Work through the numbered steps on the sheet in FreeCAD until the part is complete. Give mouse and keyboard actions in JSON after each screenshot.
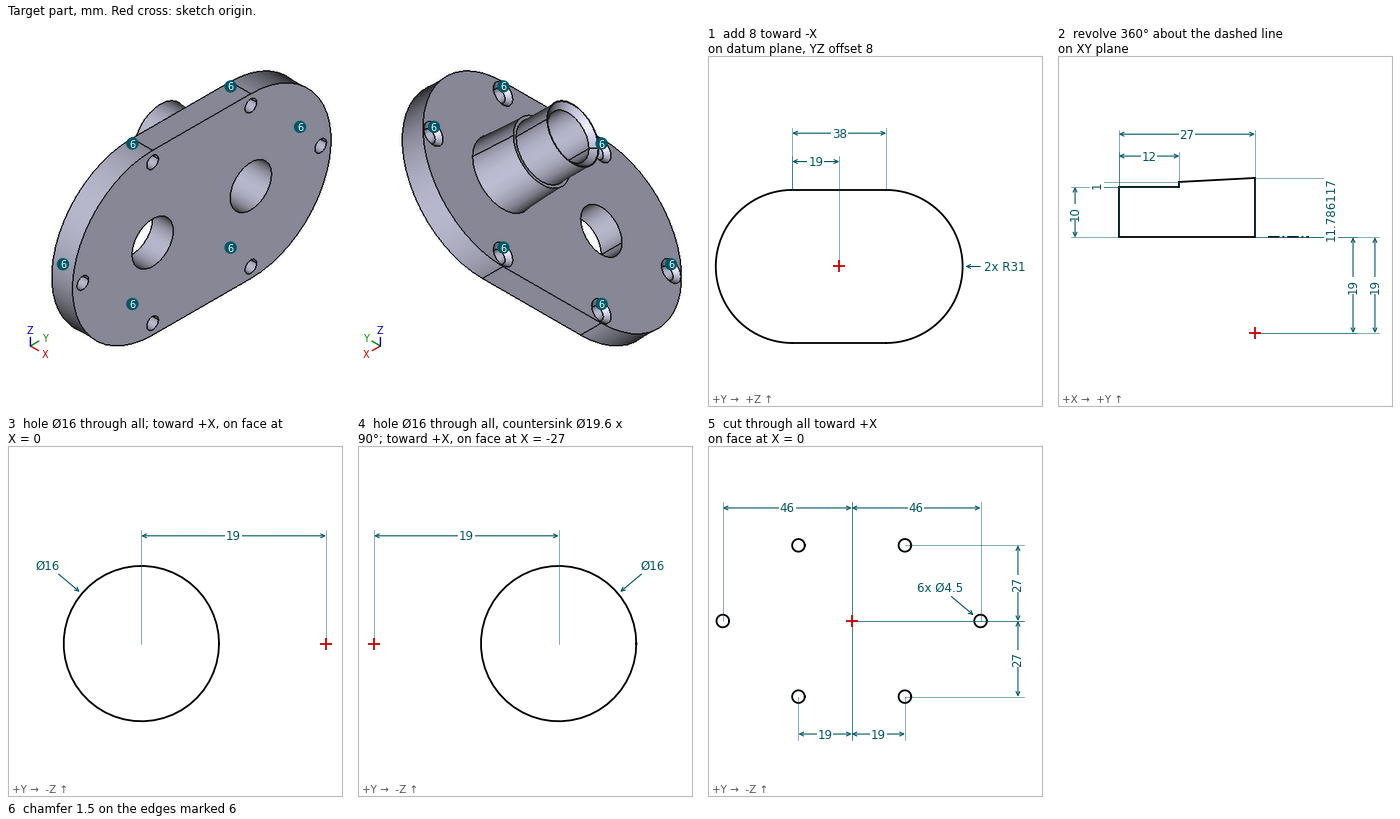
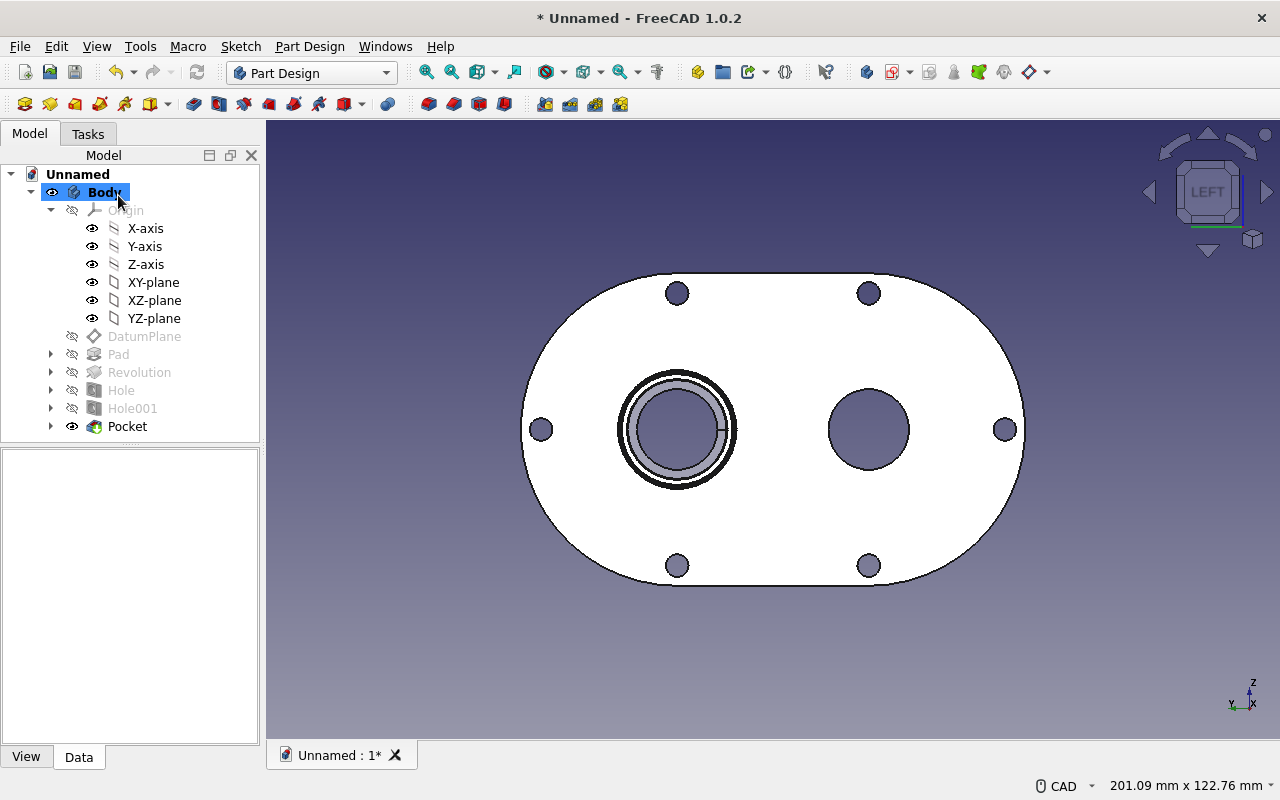
{"action": "left_click", "coordinate": [1016, 428]}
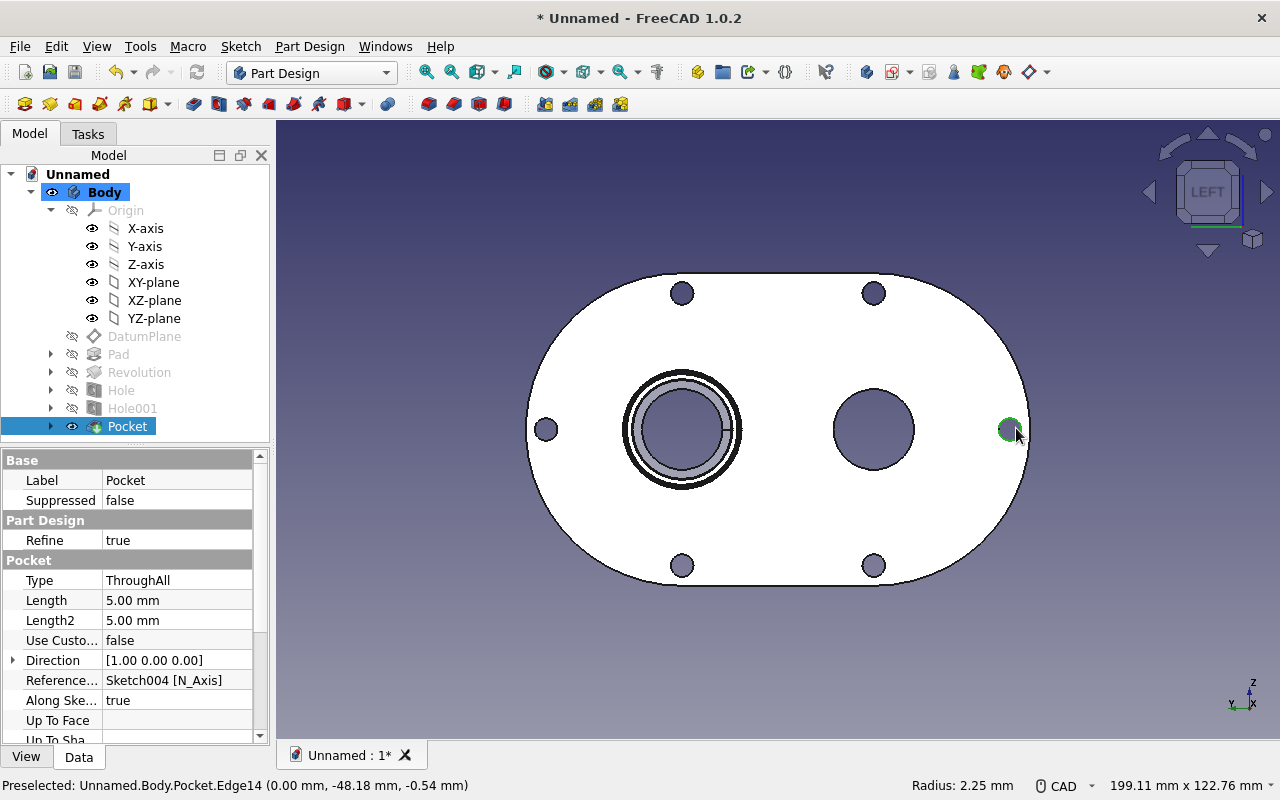
{"action": "left_click", "coordinate": [885, 565], "text": "ctrl"}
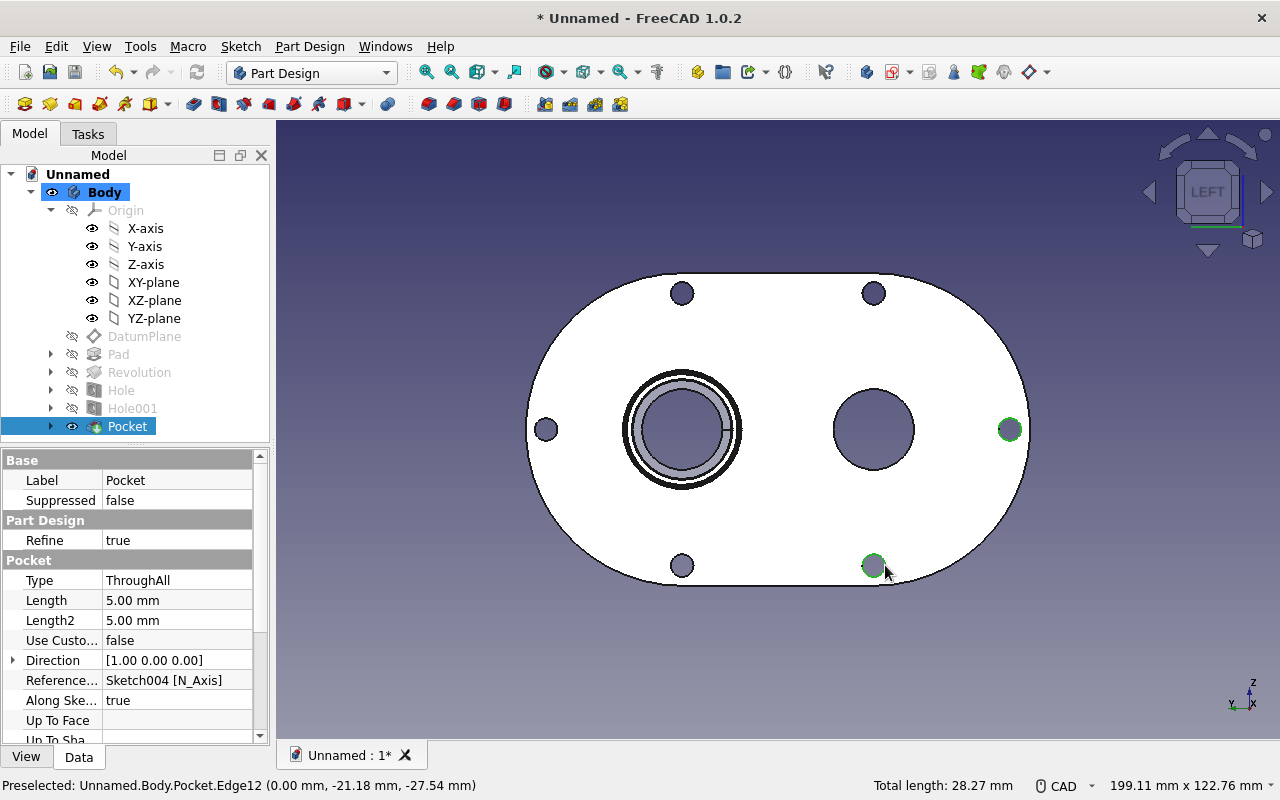
{"action": "left_click", "coordinate": [885, 292], "text": "ctrl"}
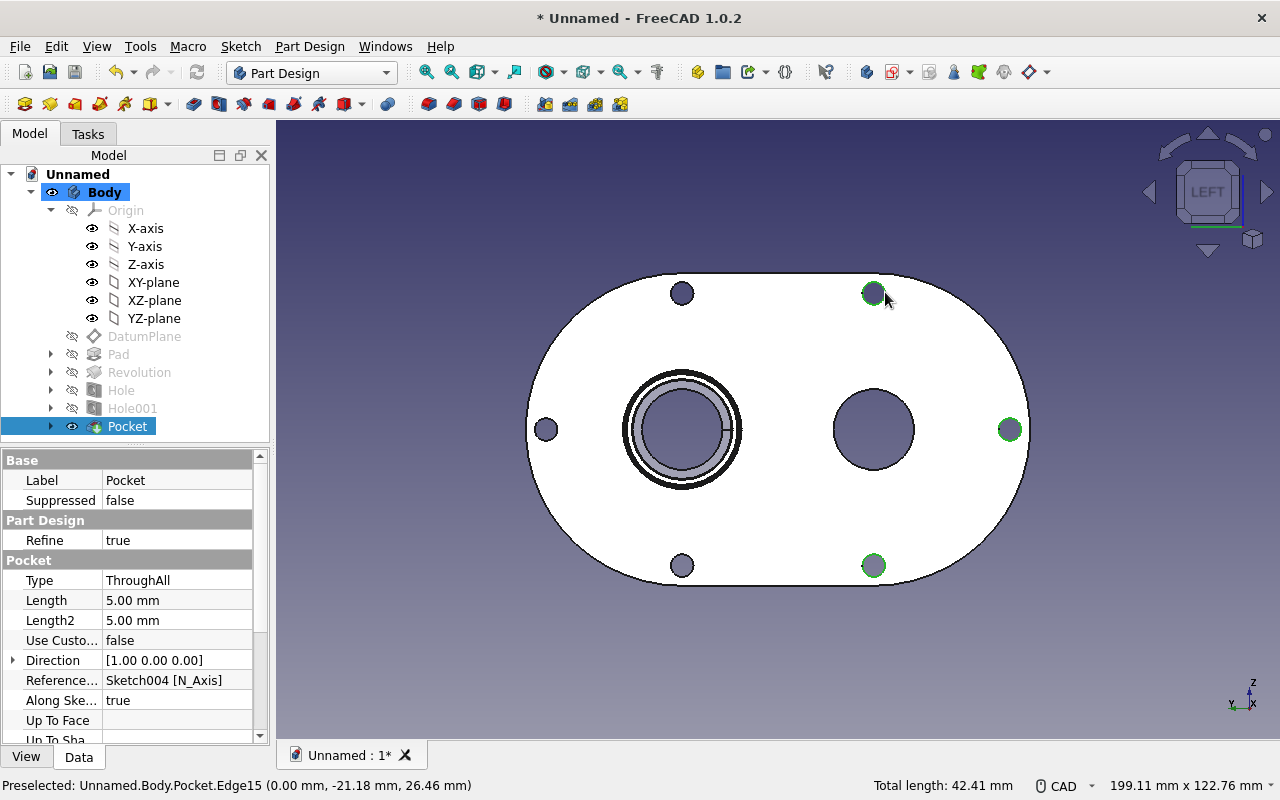
{"action": "left_click", "coordinate": [694, 565], "text": "ctrl"}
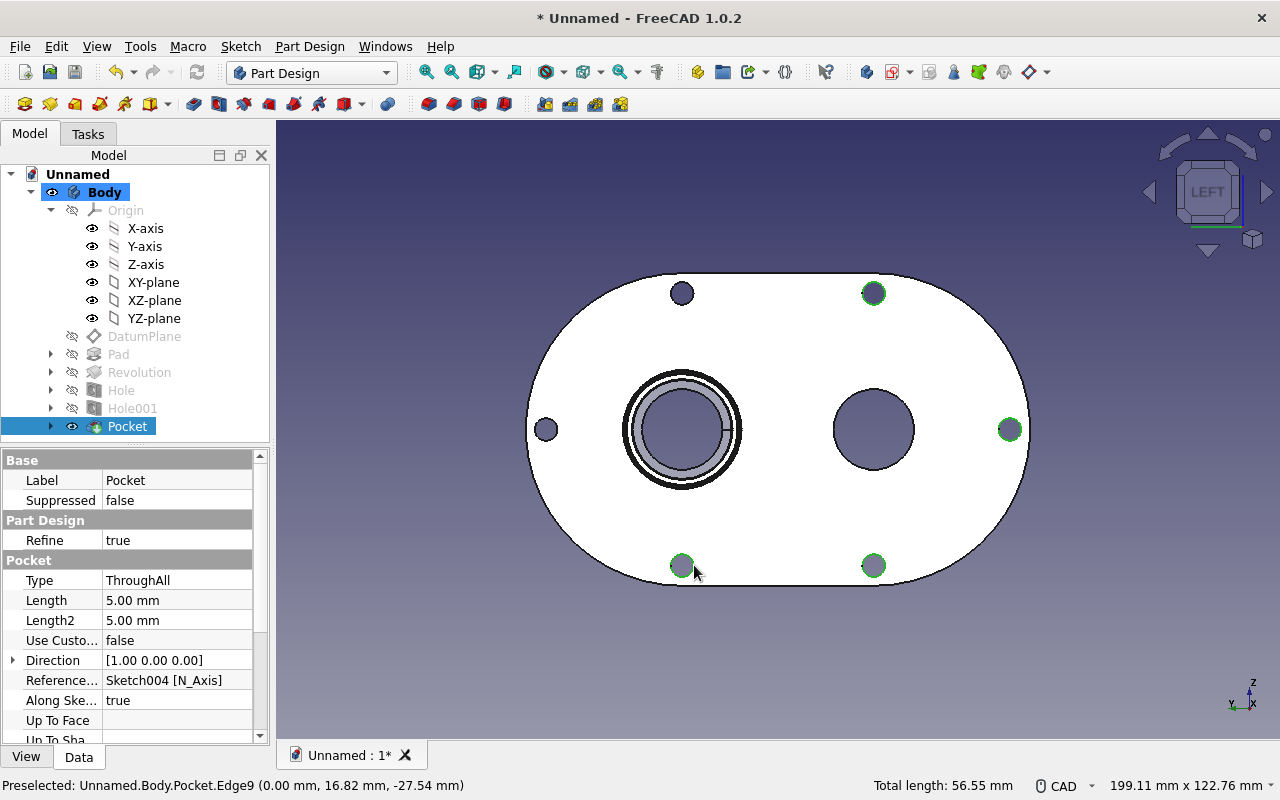
{"action": "left_click", "coordinate": [694, 292], "text": "ctrl"}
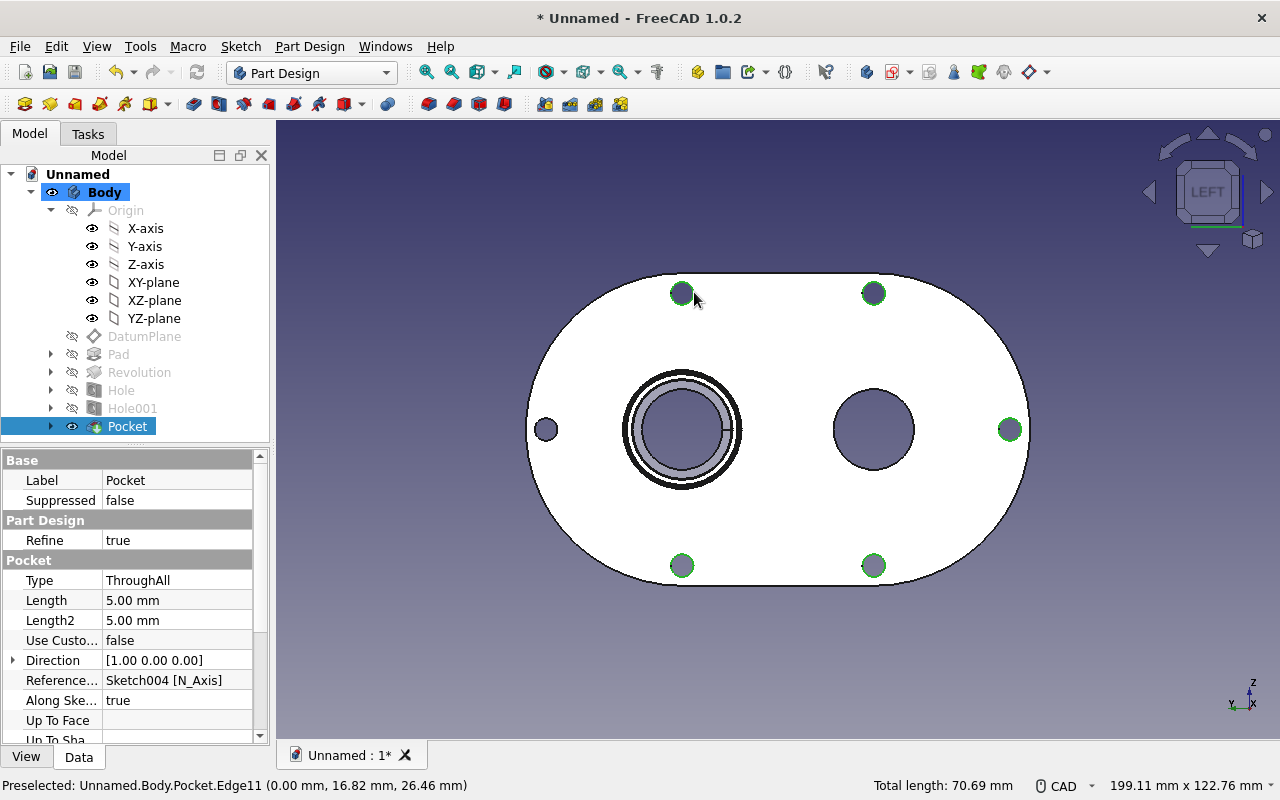
{"action": "left_click", "coordinate": [557, 428], "text": "ctrl"}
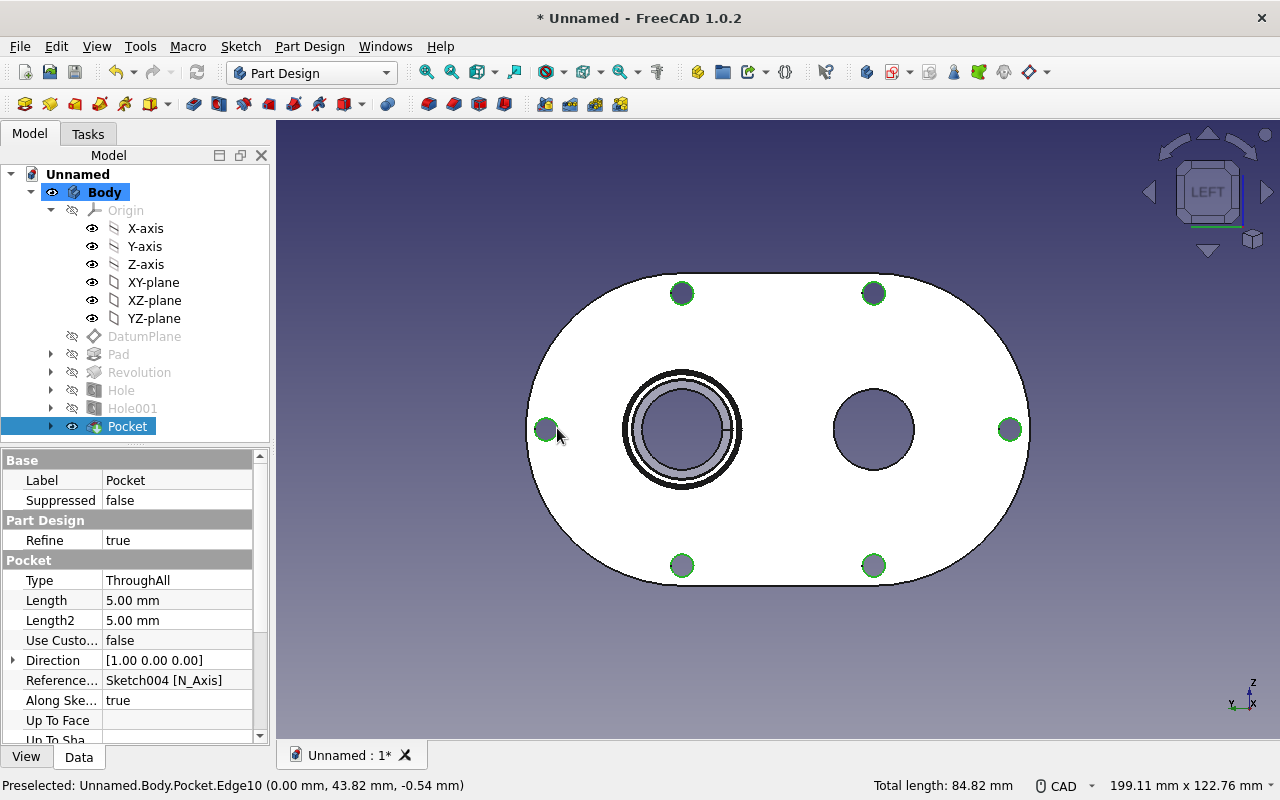
{"action": "left_click", "coordinate": [454, 104]}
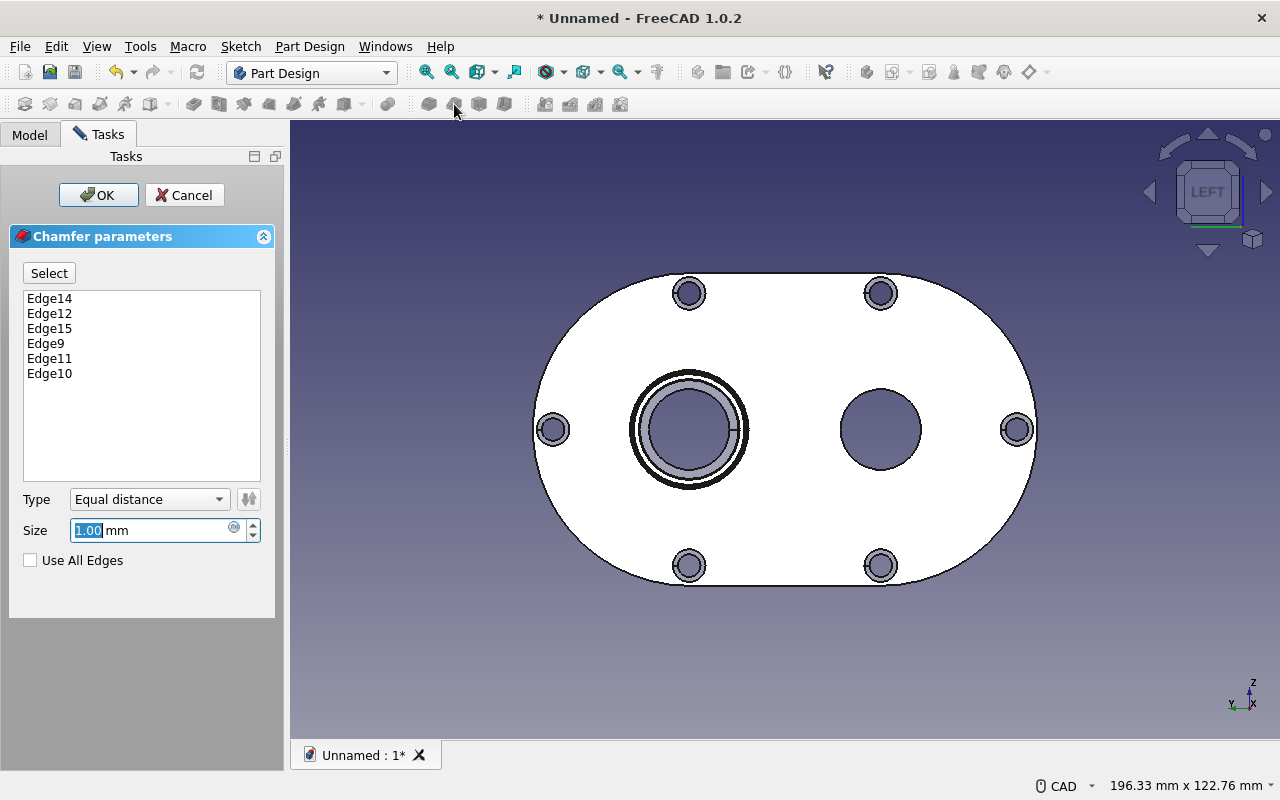
{"action": "type", "text": "1.5"}
{"action": "key", "text": "Tab"}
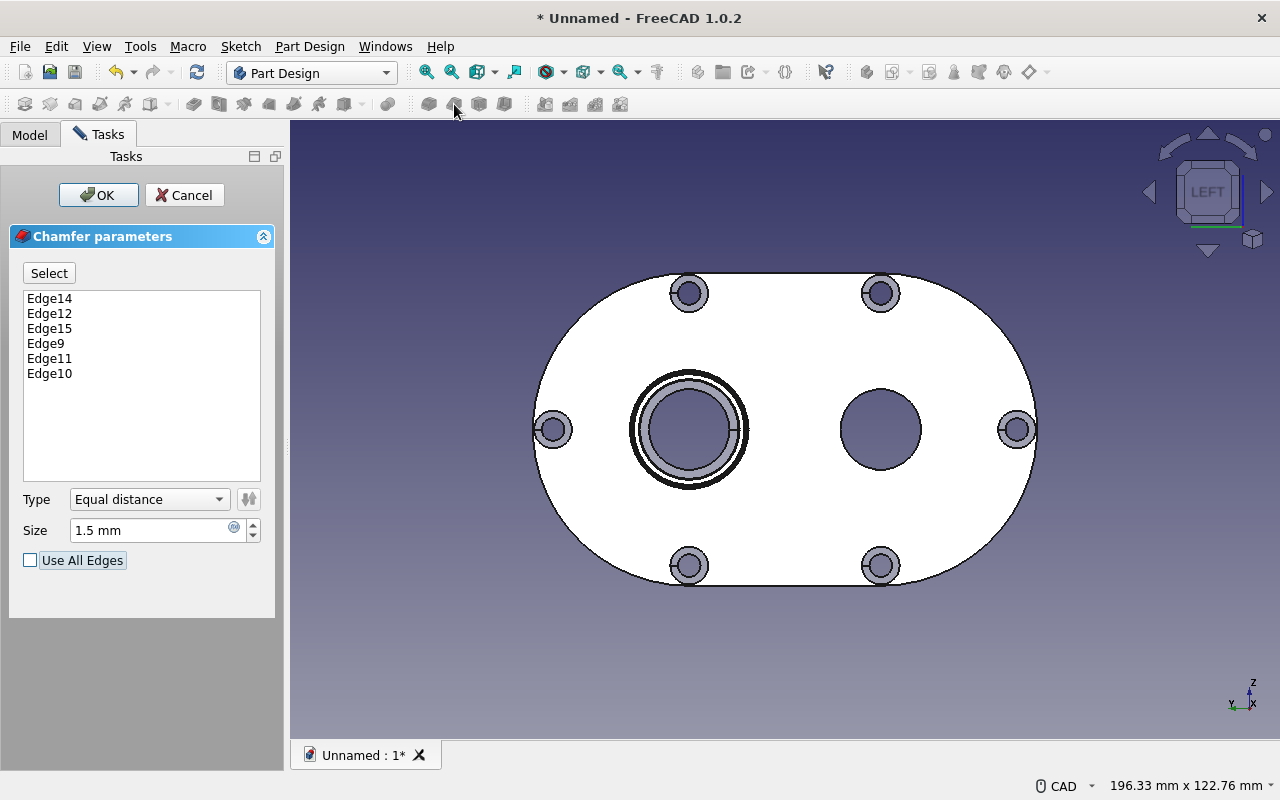
{"action": "left_click", "coordinate": [99, 195]}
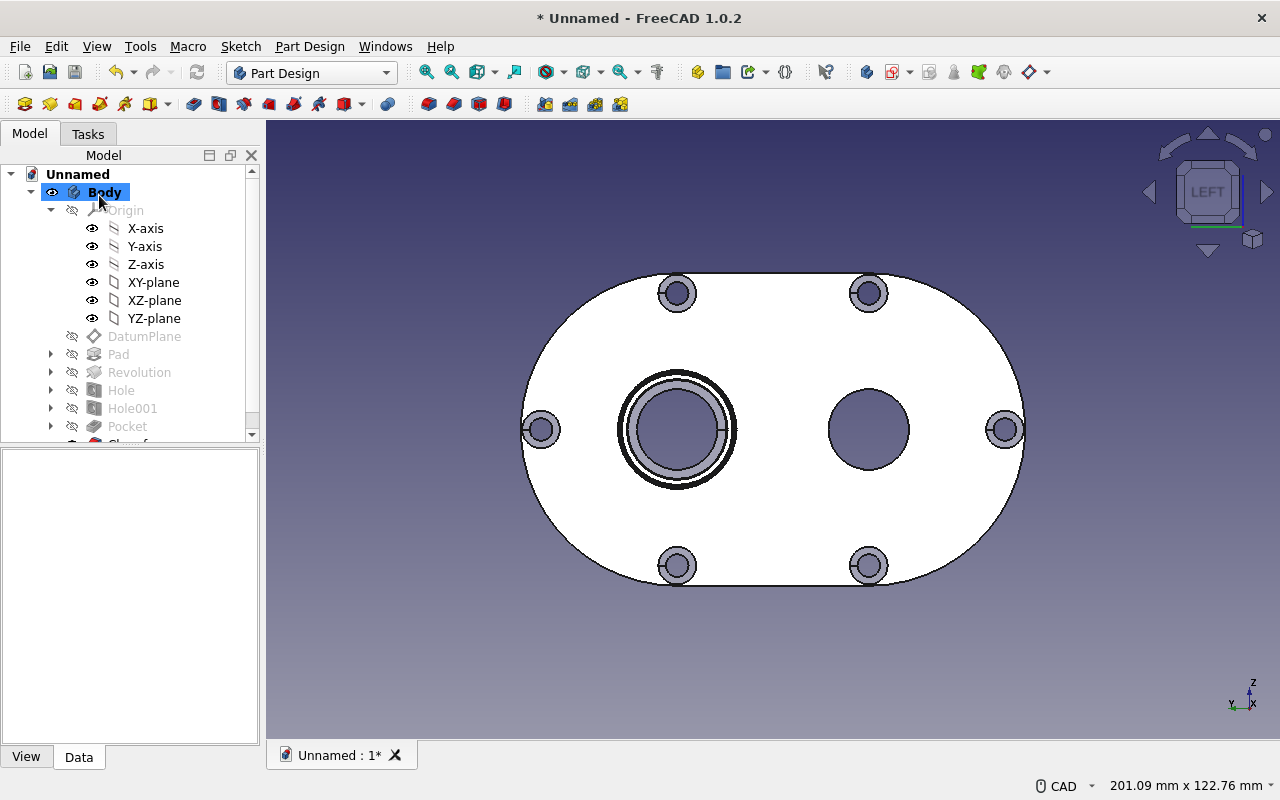
{"action": "key", "text": "0"}